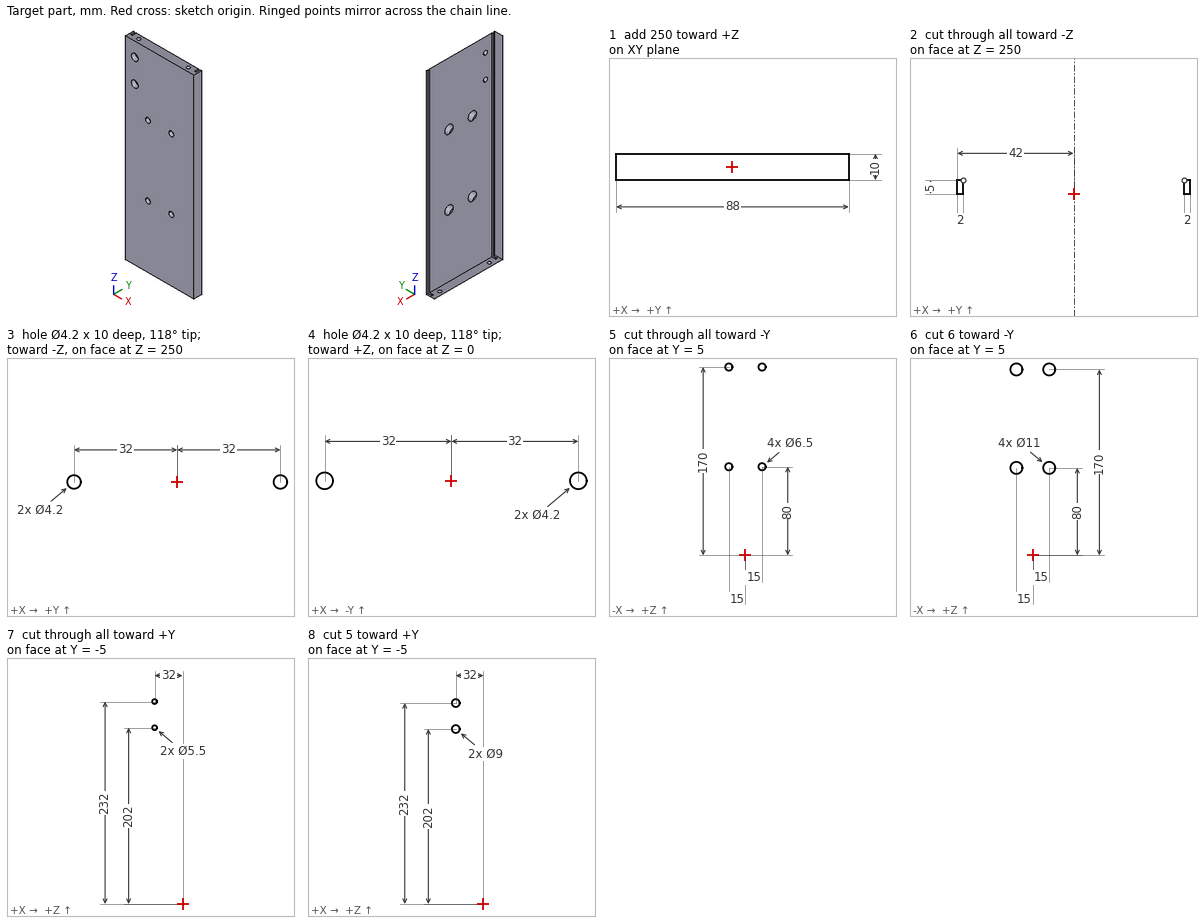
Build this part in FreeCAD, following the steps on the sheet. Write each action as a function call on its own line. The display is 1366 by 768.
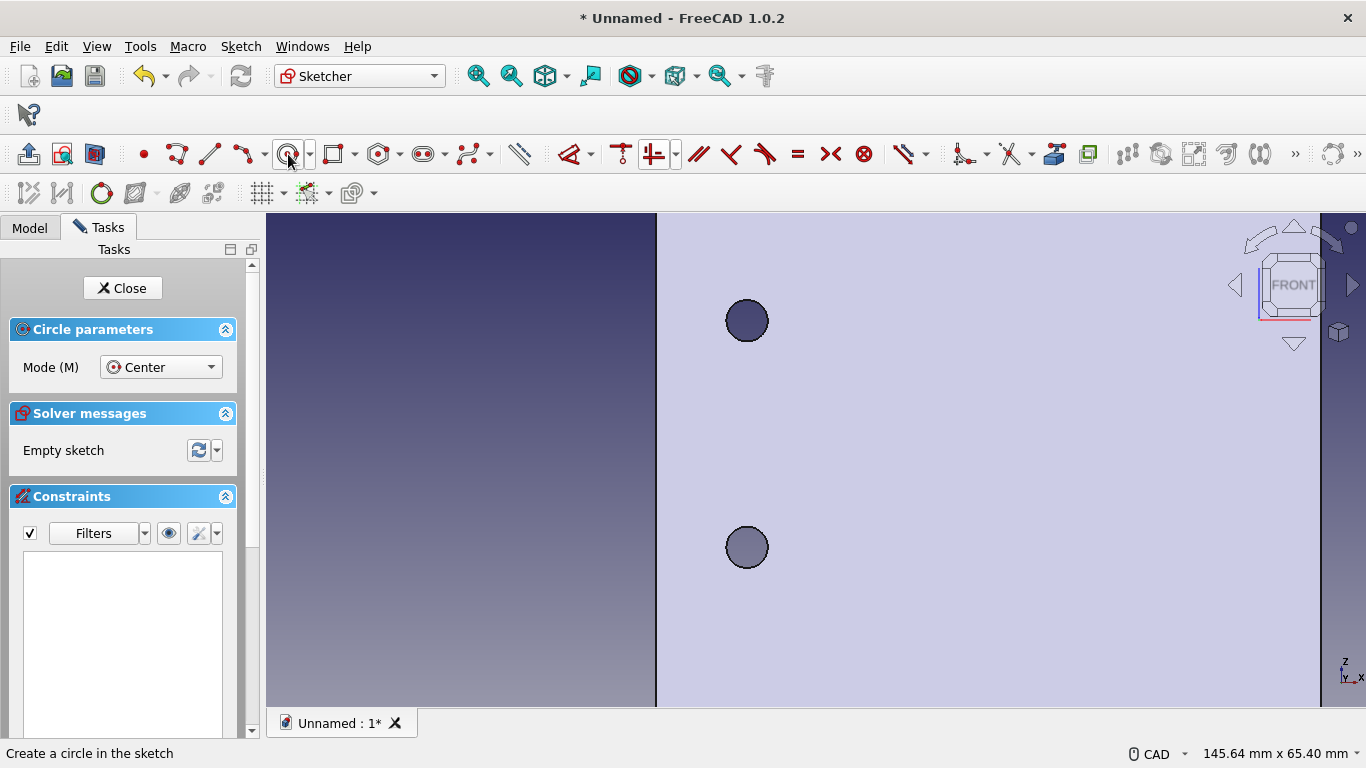
click(747, 321)
move(771, 297)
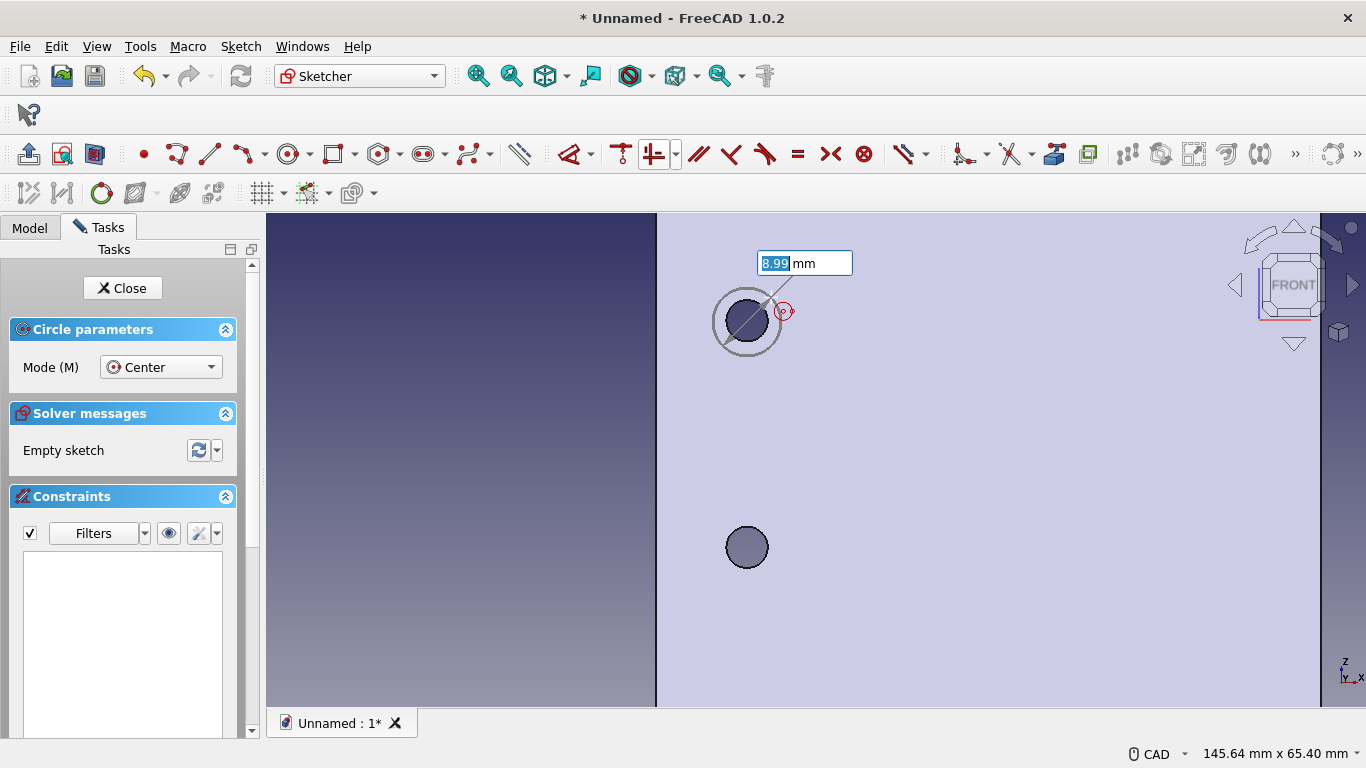
text(9)
key(Return)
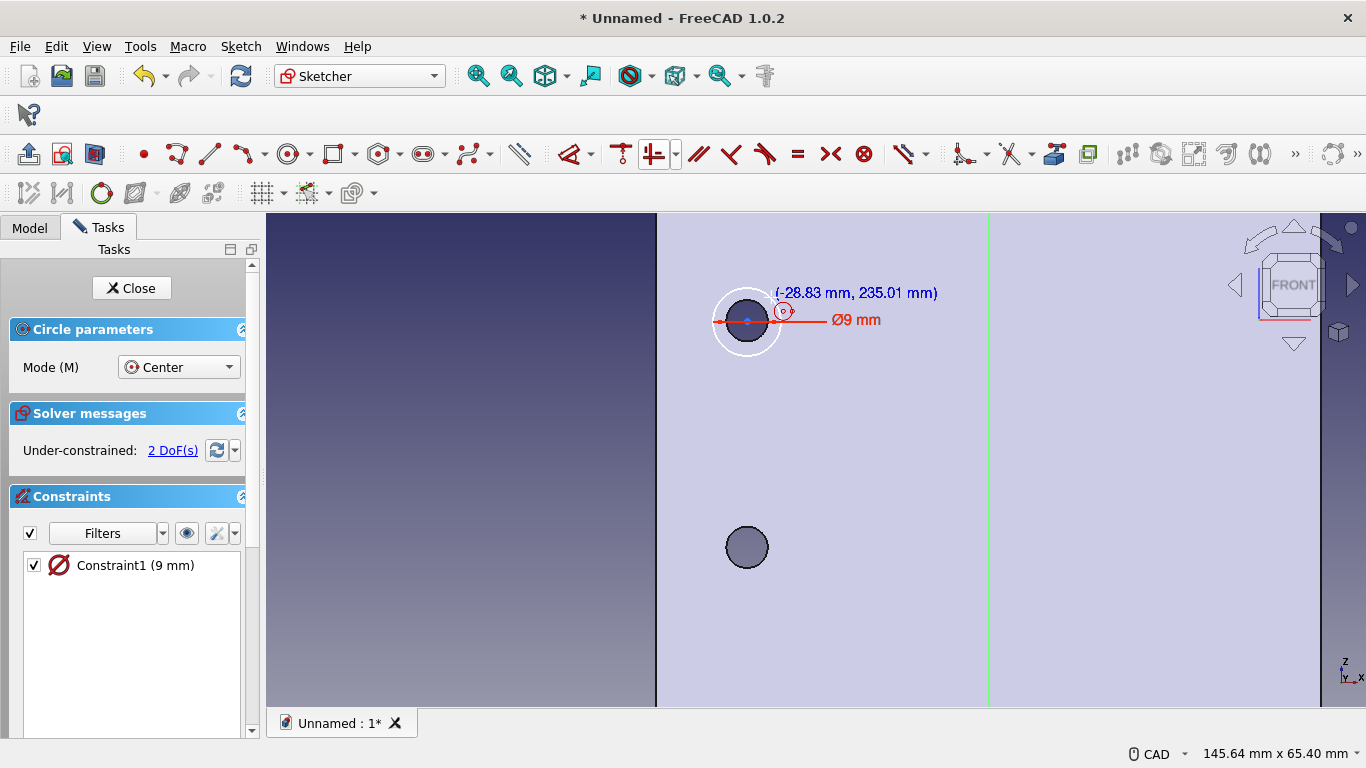
click(747, 547)
move(771, 523)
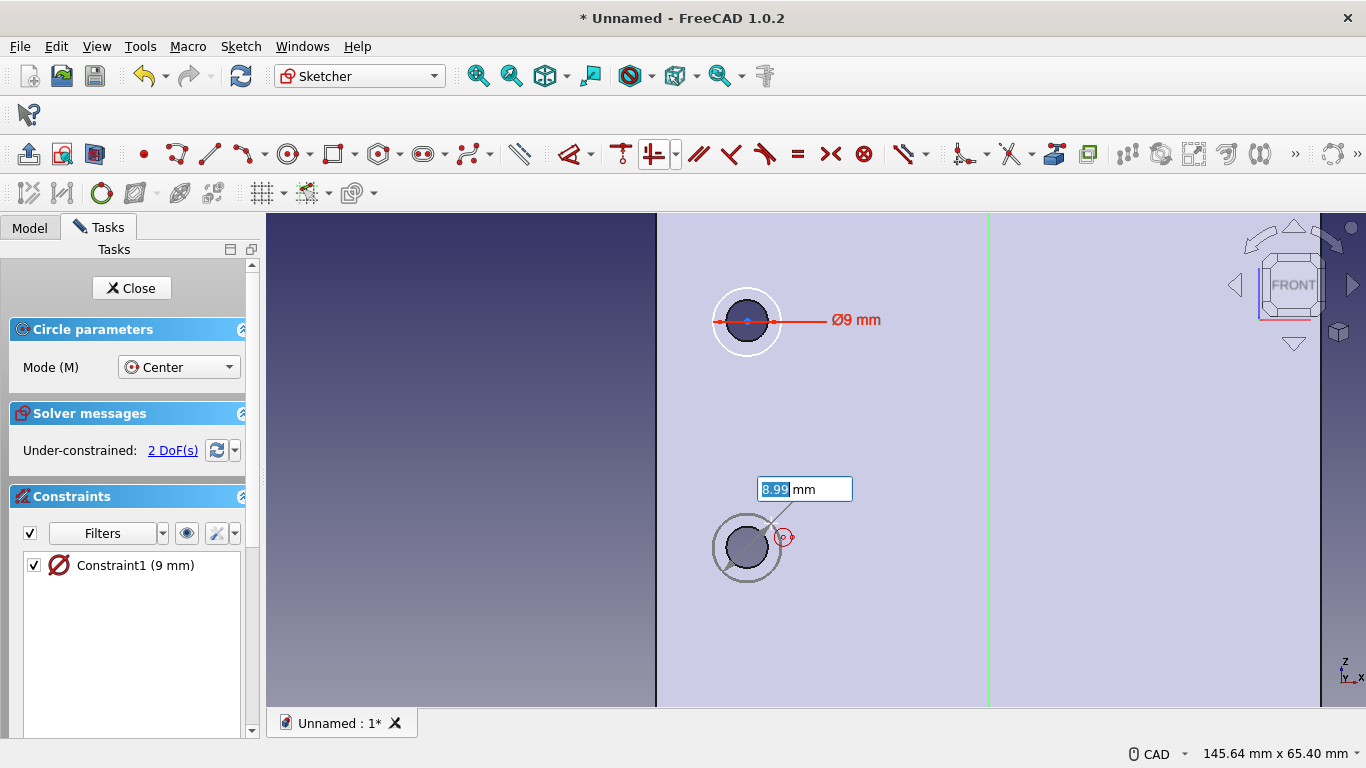
text(9)
key(Return)
key(Escape)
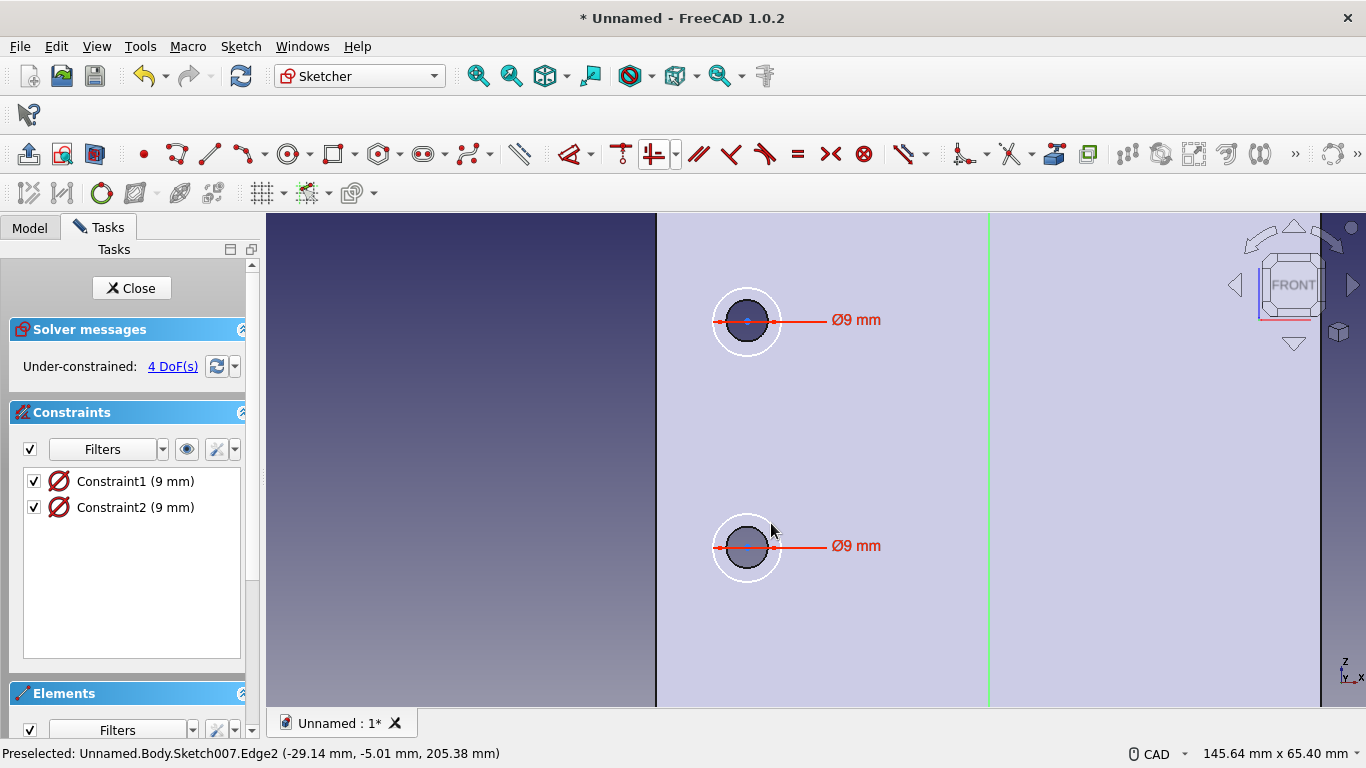
click(747, 322)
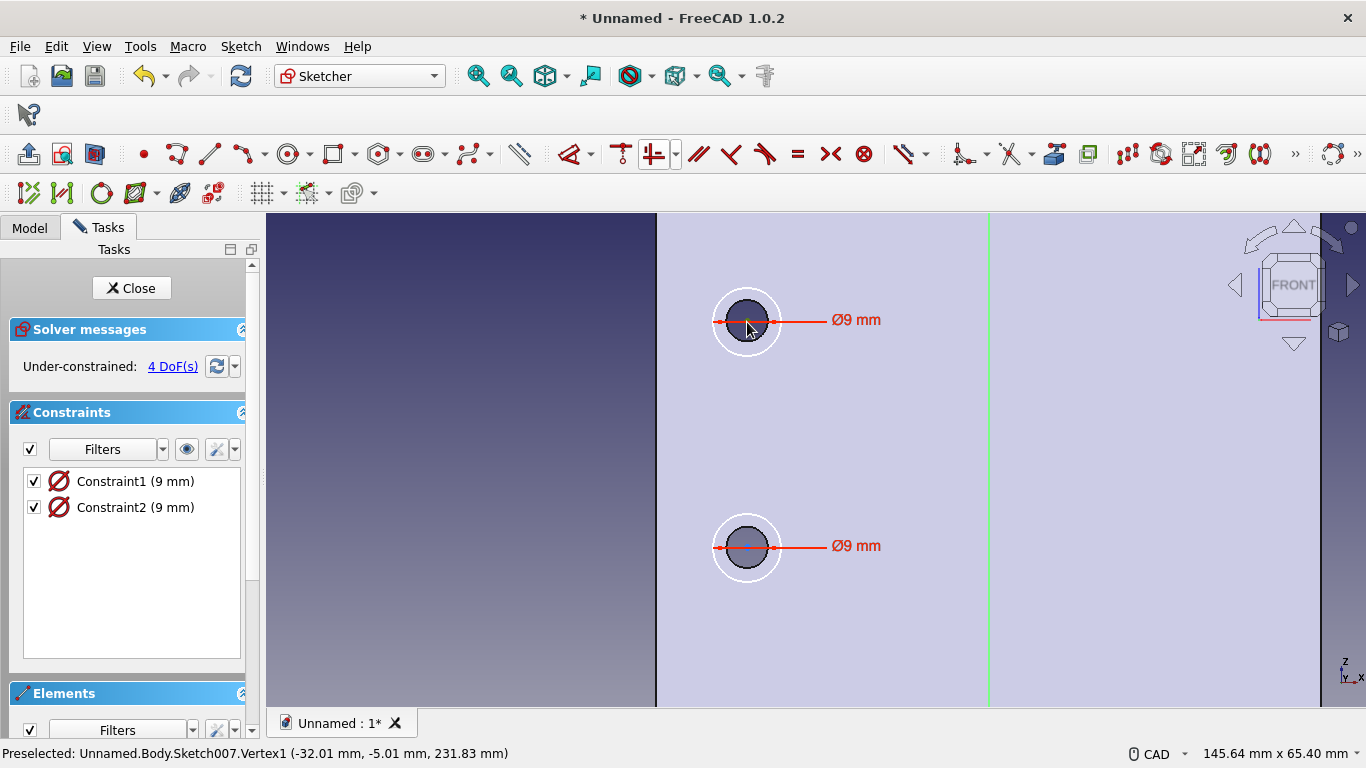
click(747, 548)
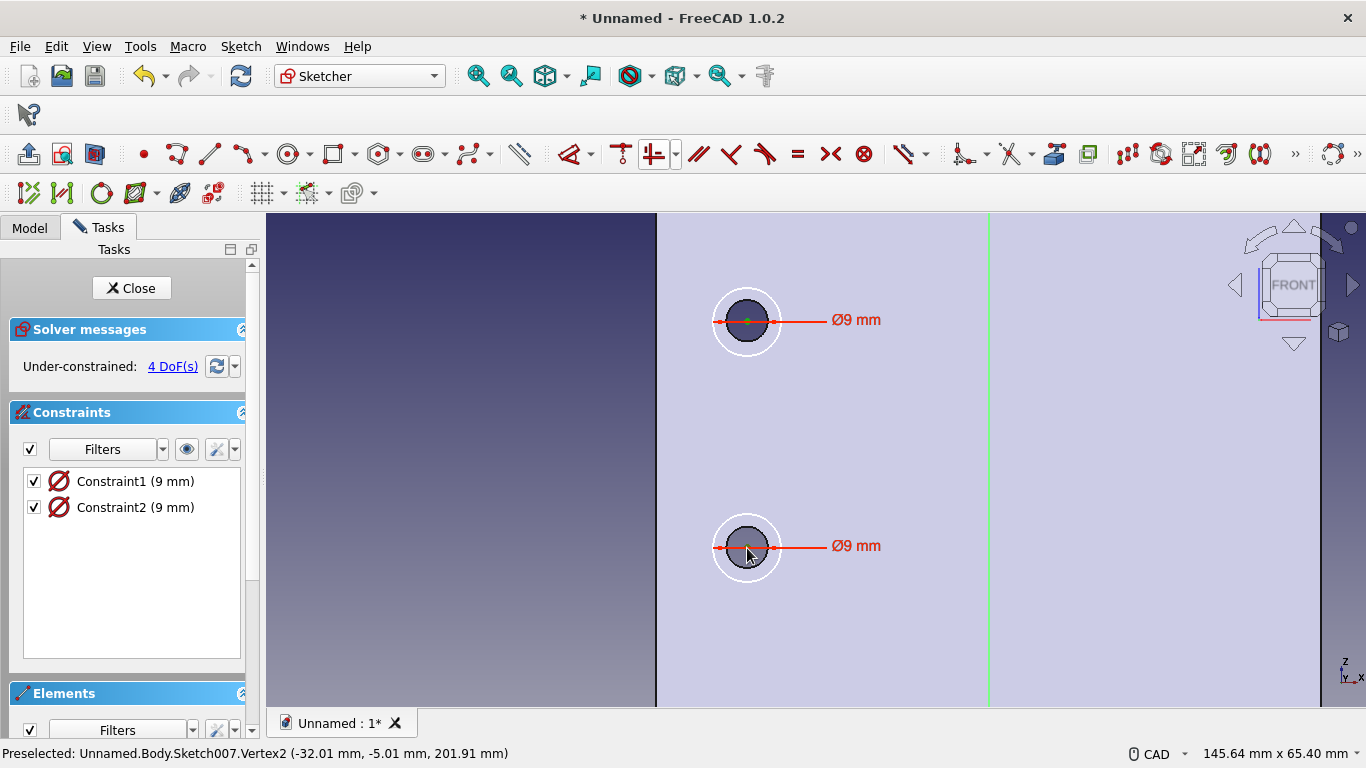
key(v)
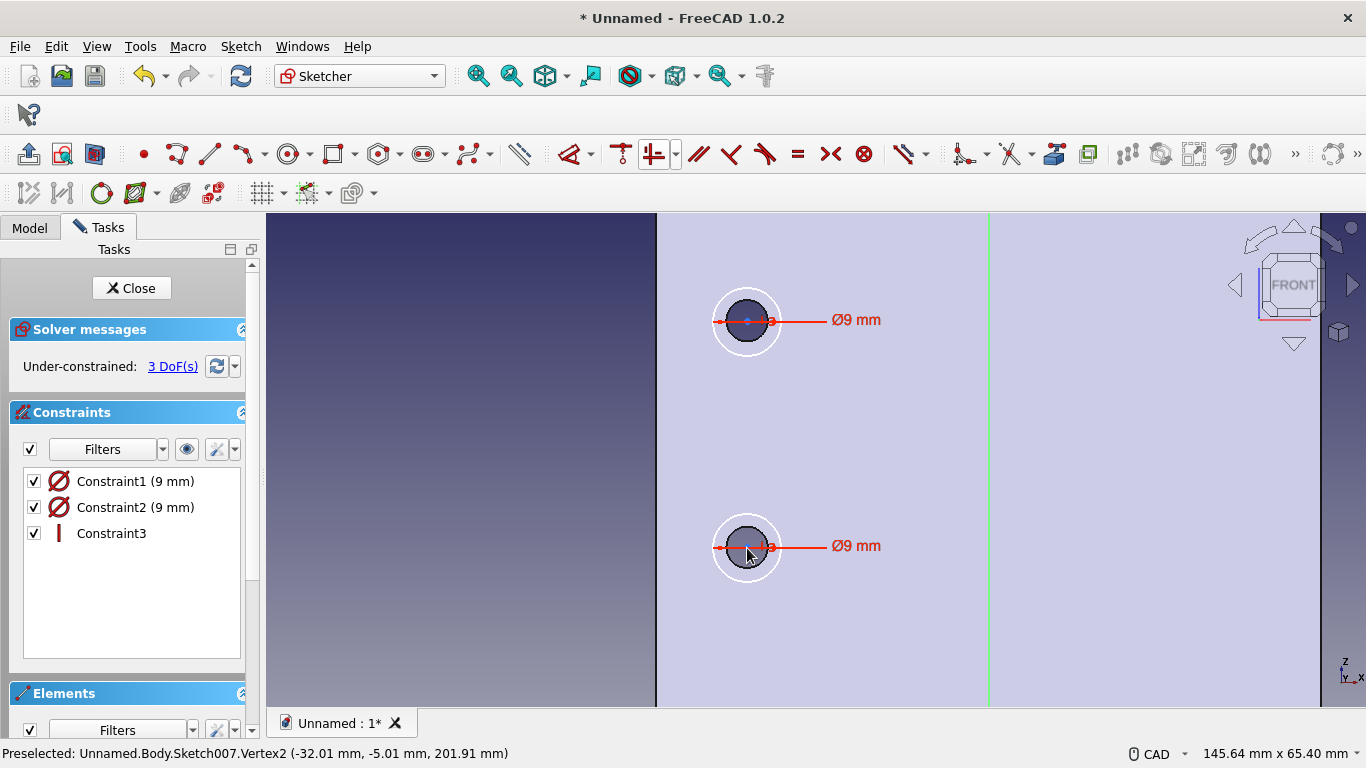
click(568, 154)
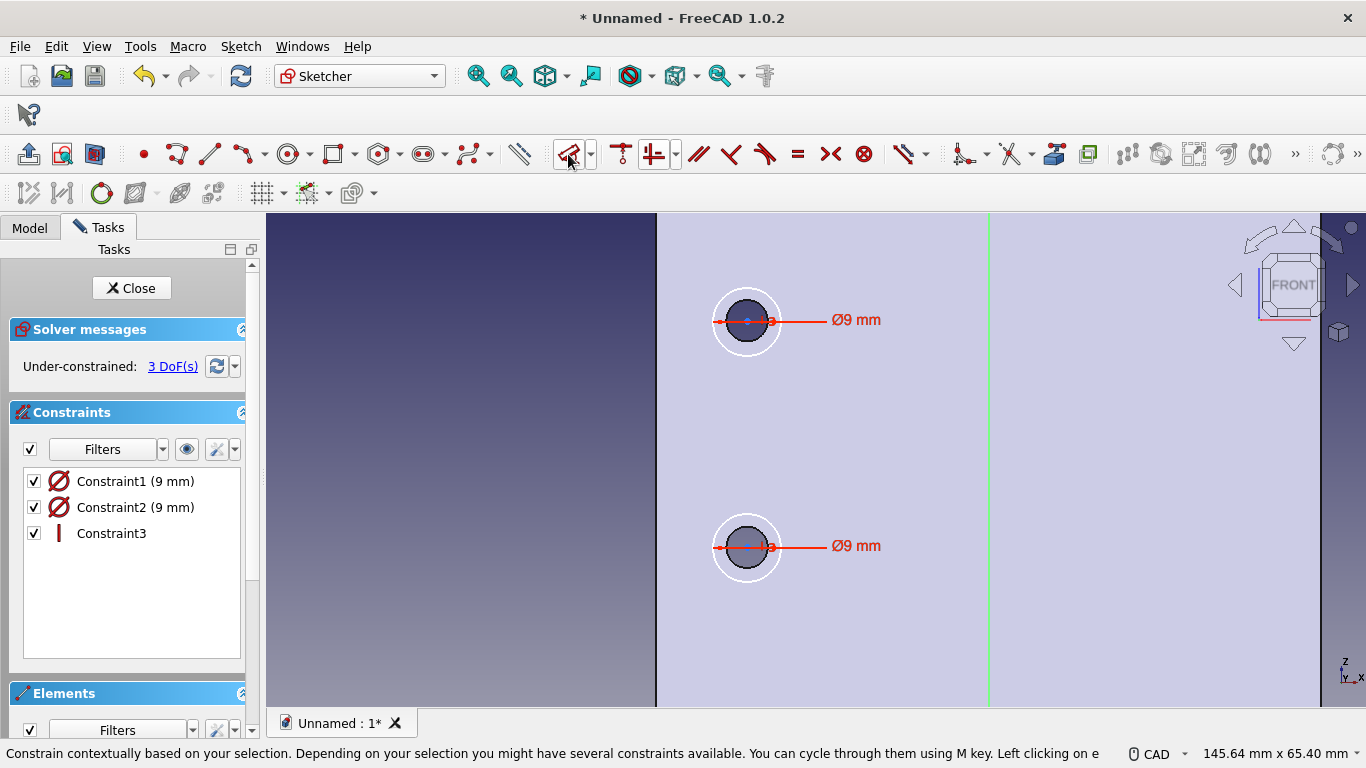
click(747, 322)
click(868, 288)